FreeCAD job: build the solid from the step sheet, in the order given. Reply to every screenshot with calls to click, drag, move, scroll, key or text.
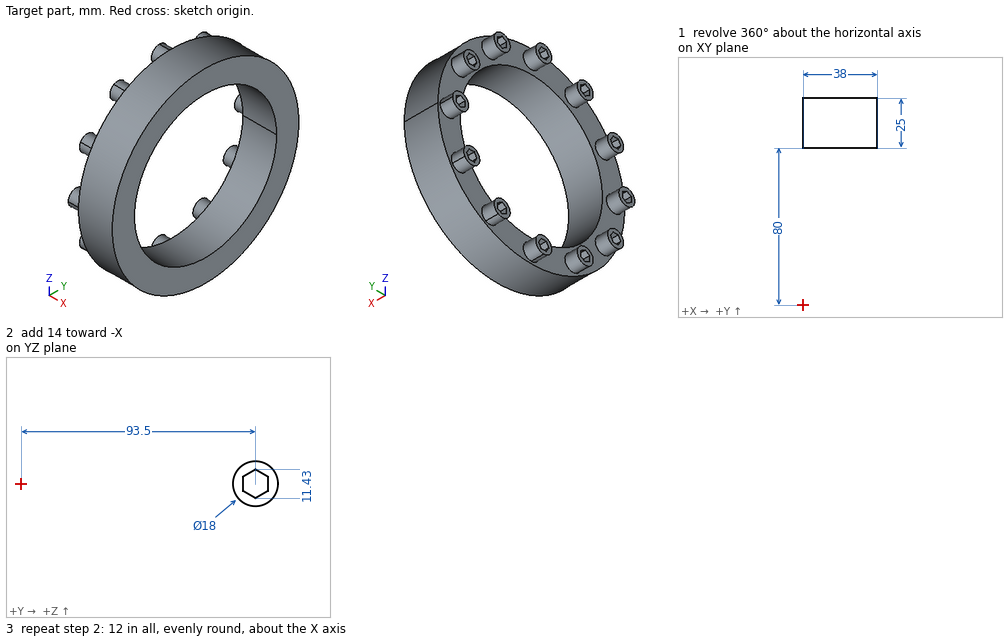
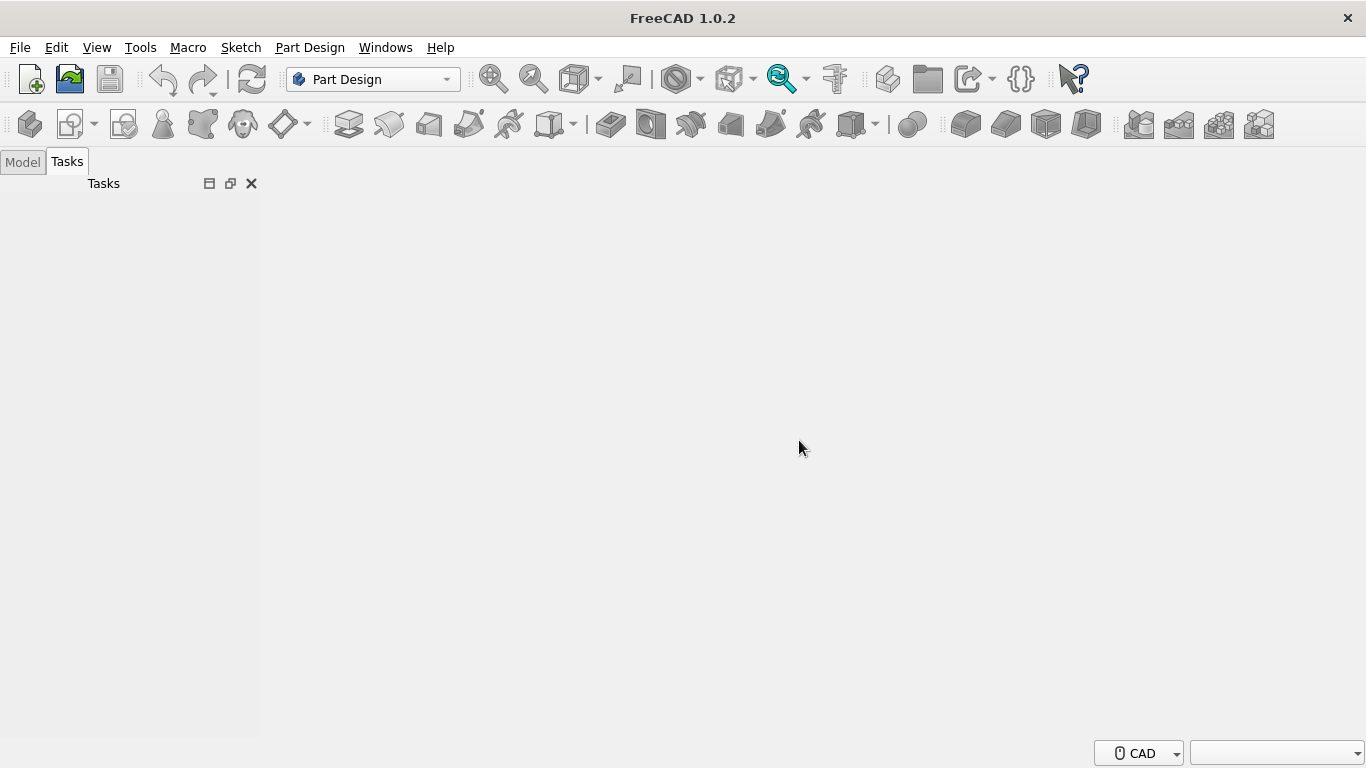
click(30, 80)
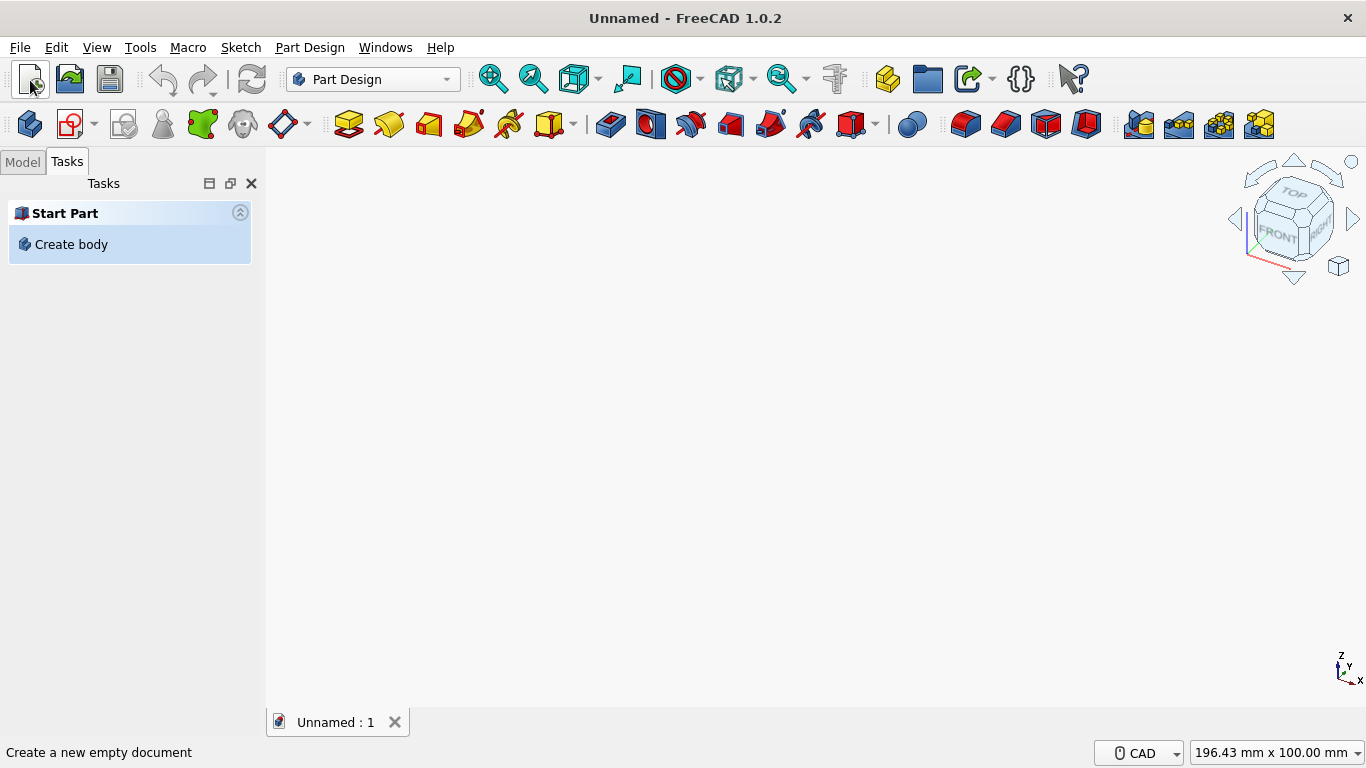
click(70, 124)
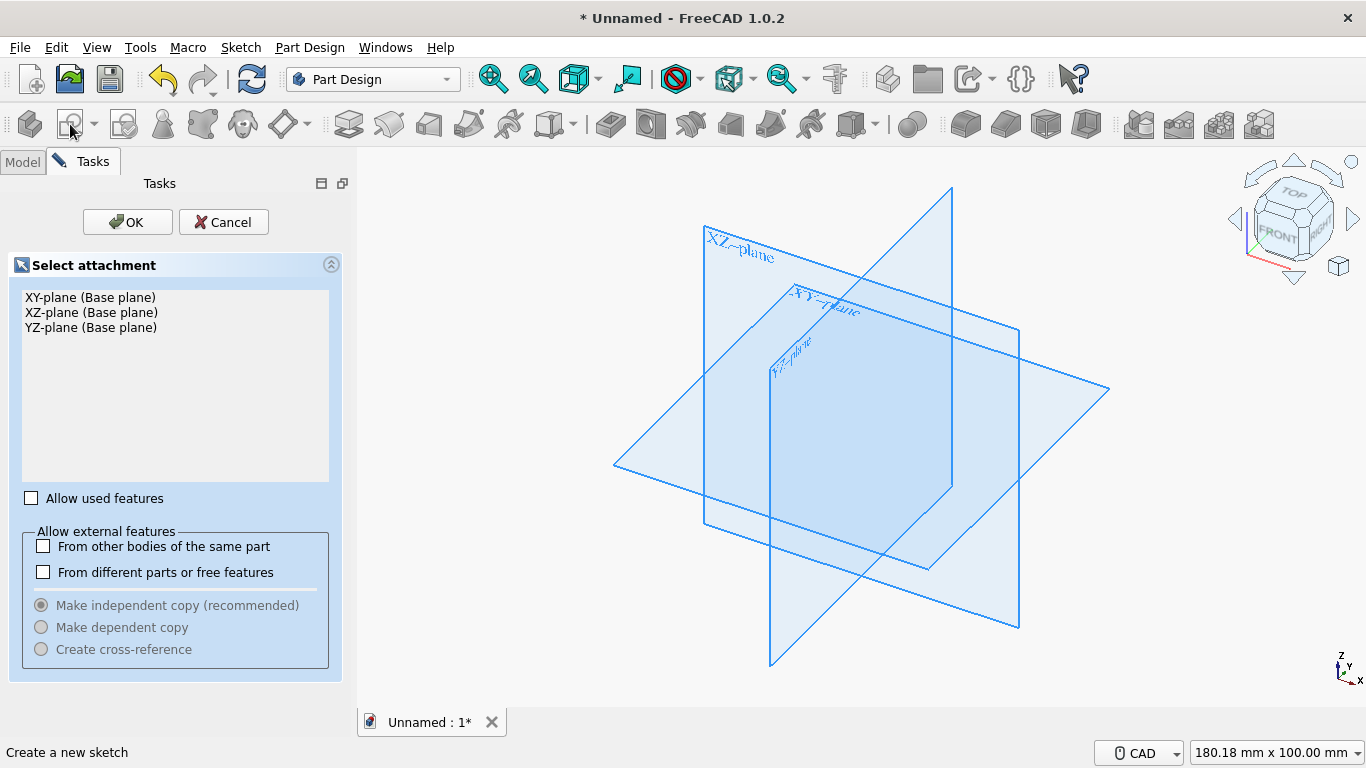
click(82, 298)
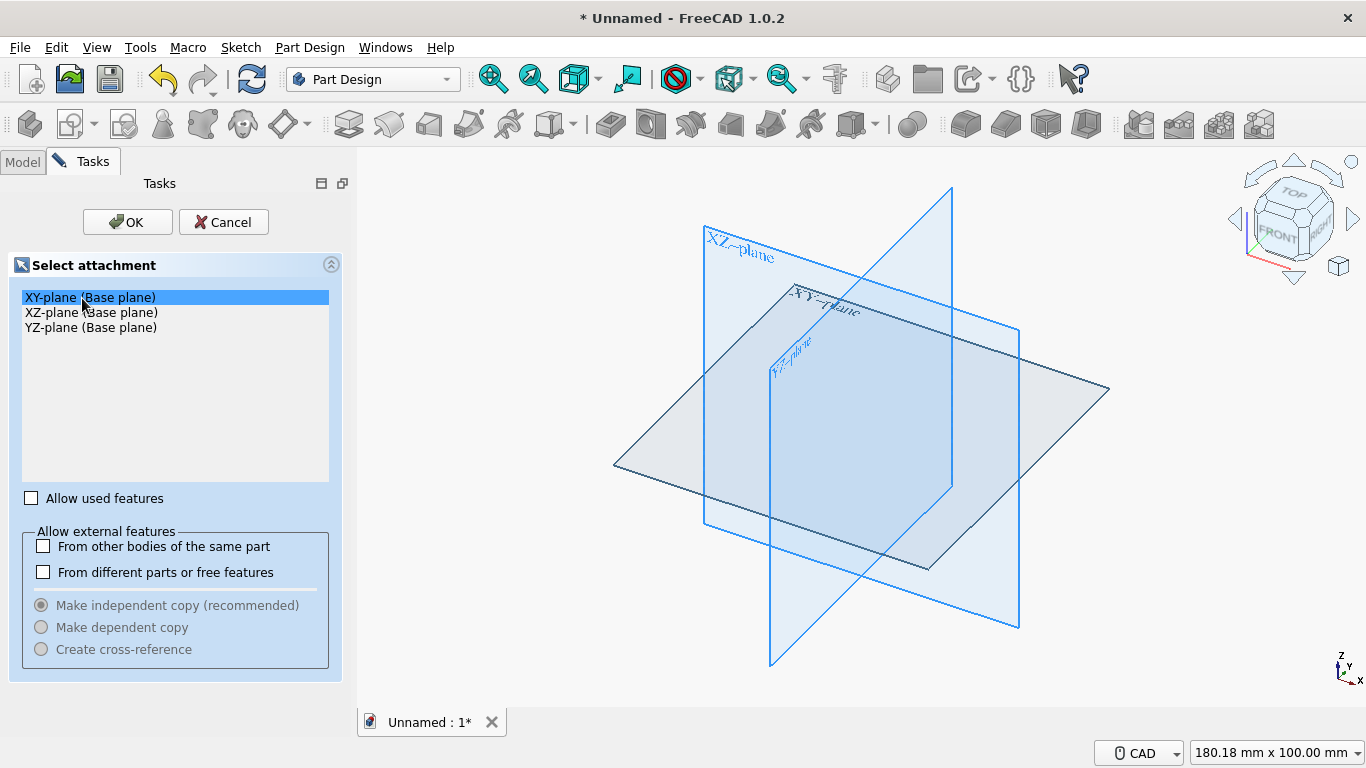
click(128, 222)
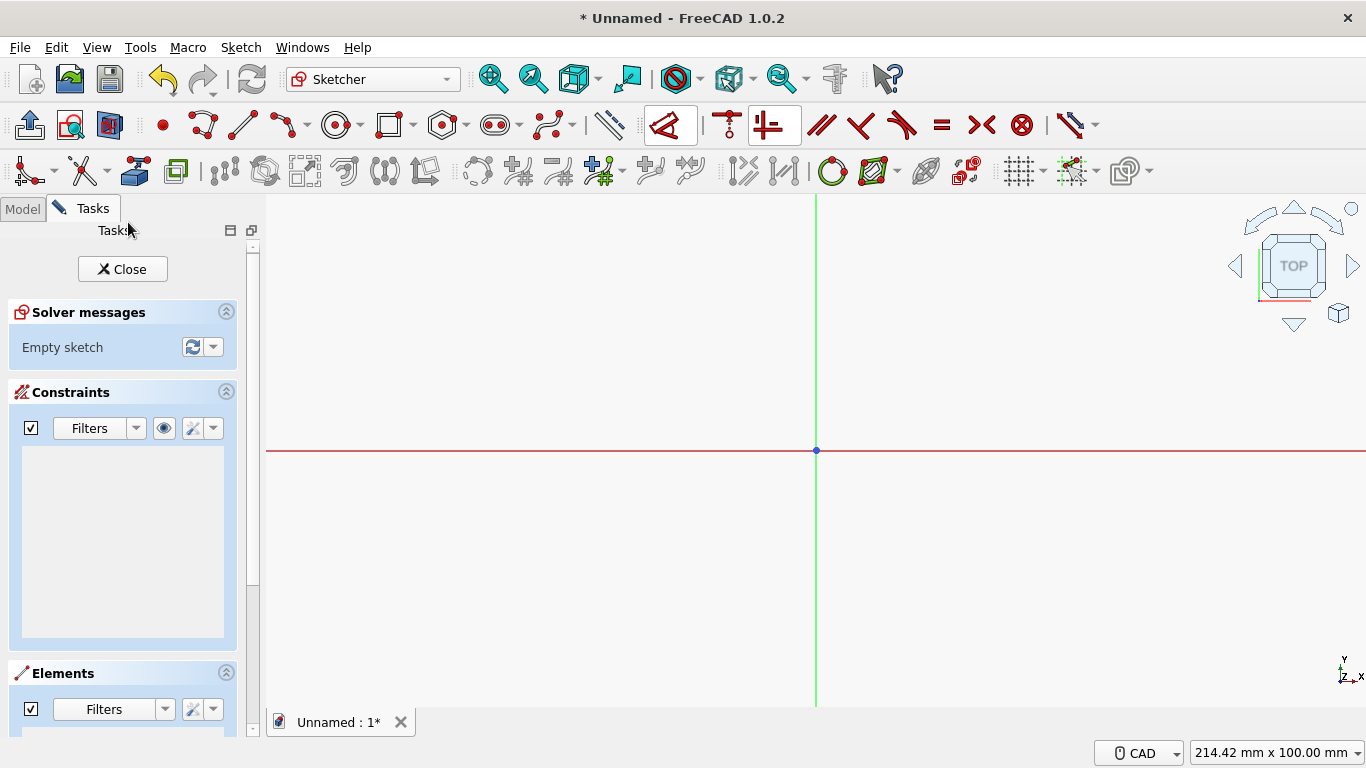
scroll(748, 450, down, 5)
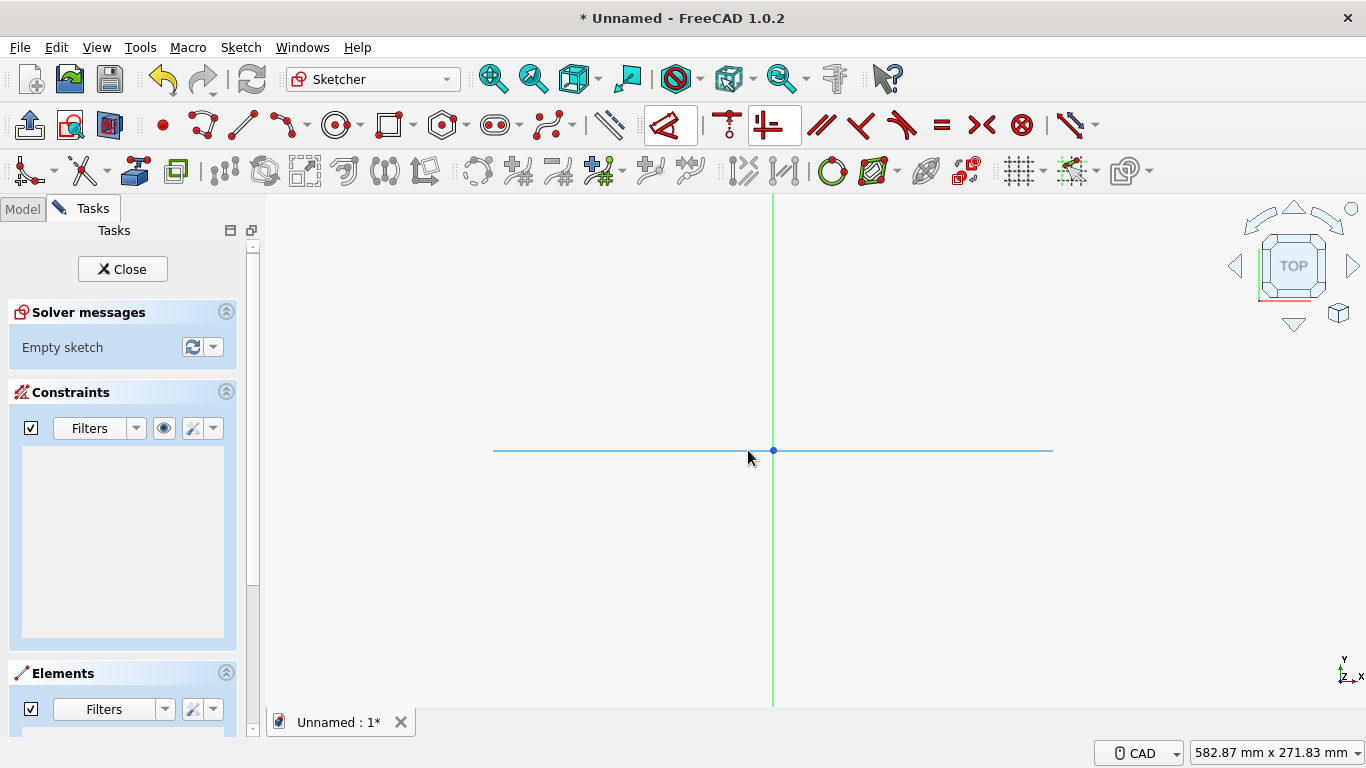
scroll(819, 249, up, 10)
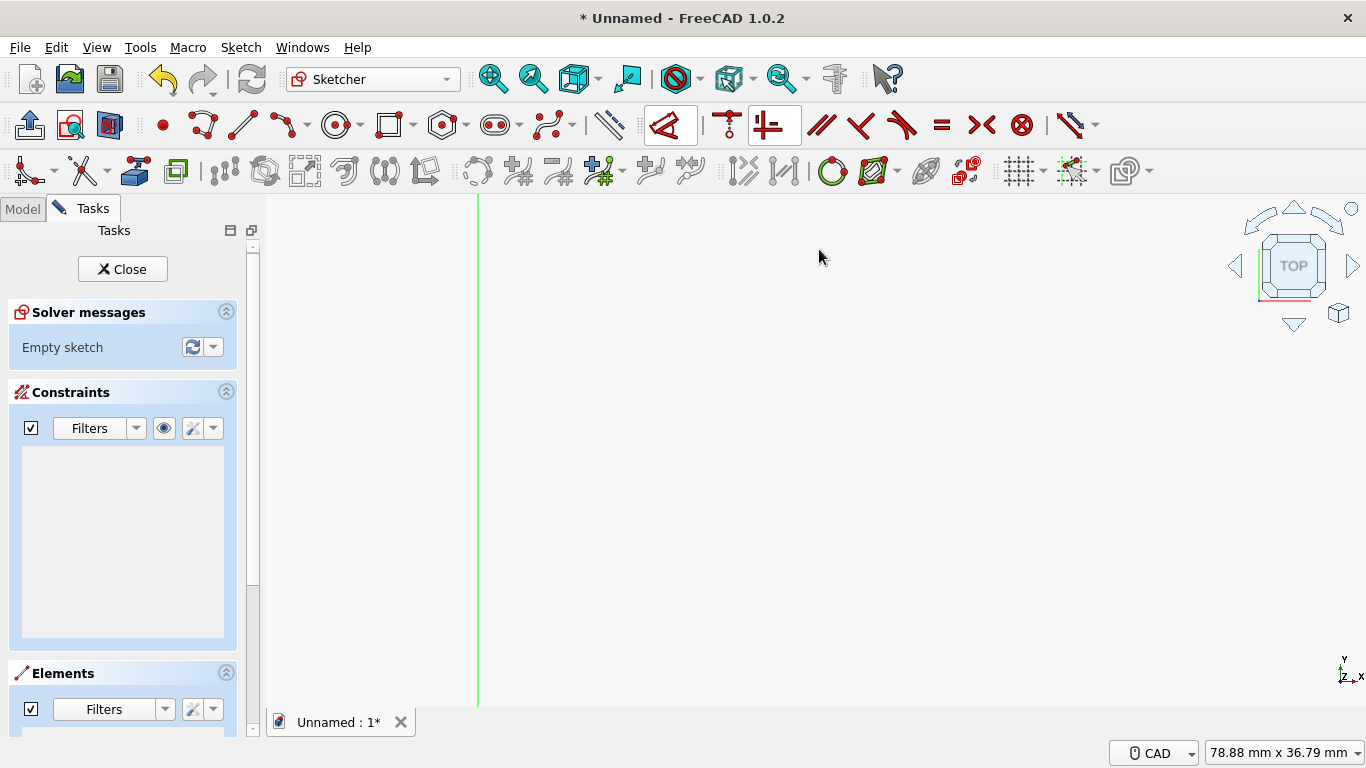
click(390, 126)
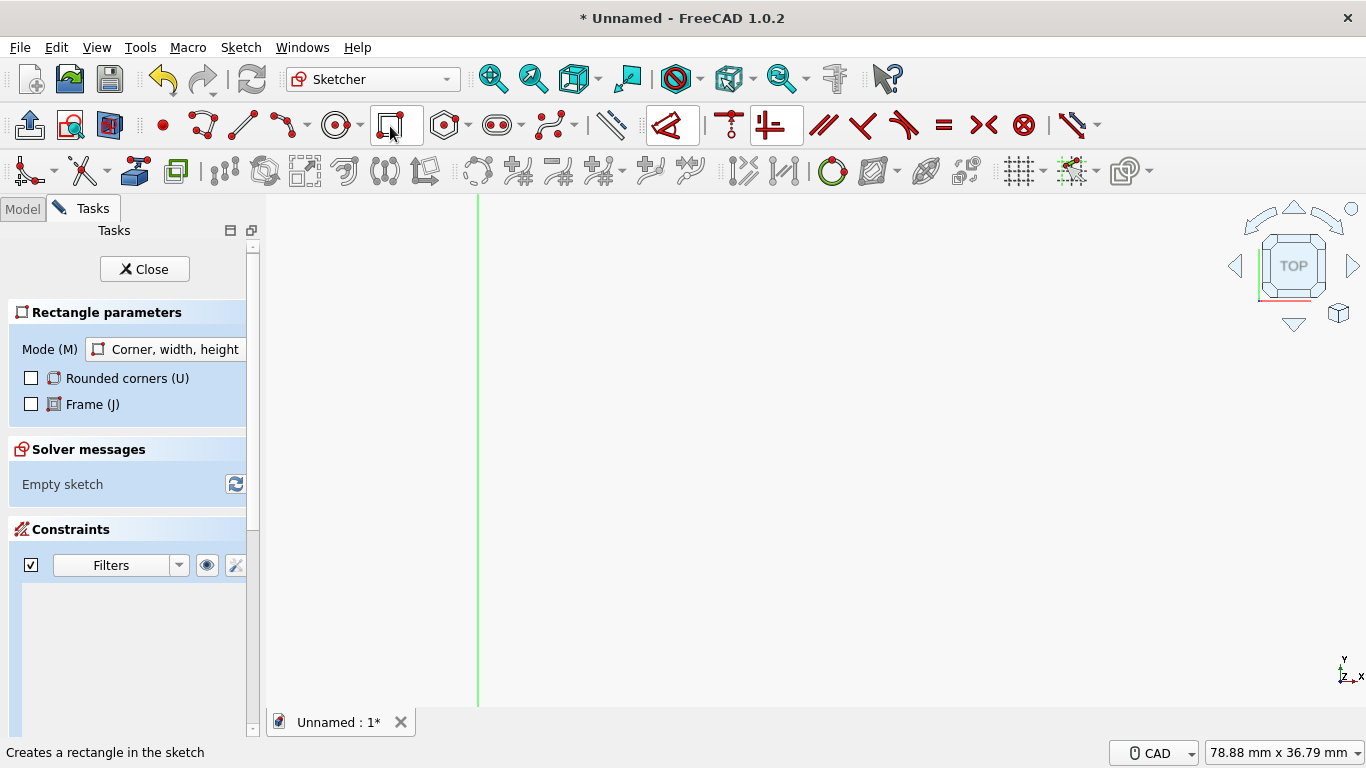
click(478, 273)
move(1008, 622)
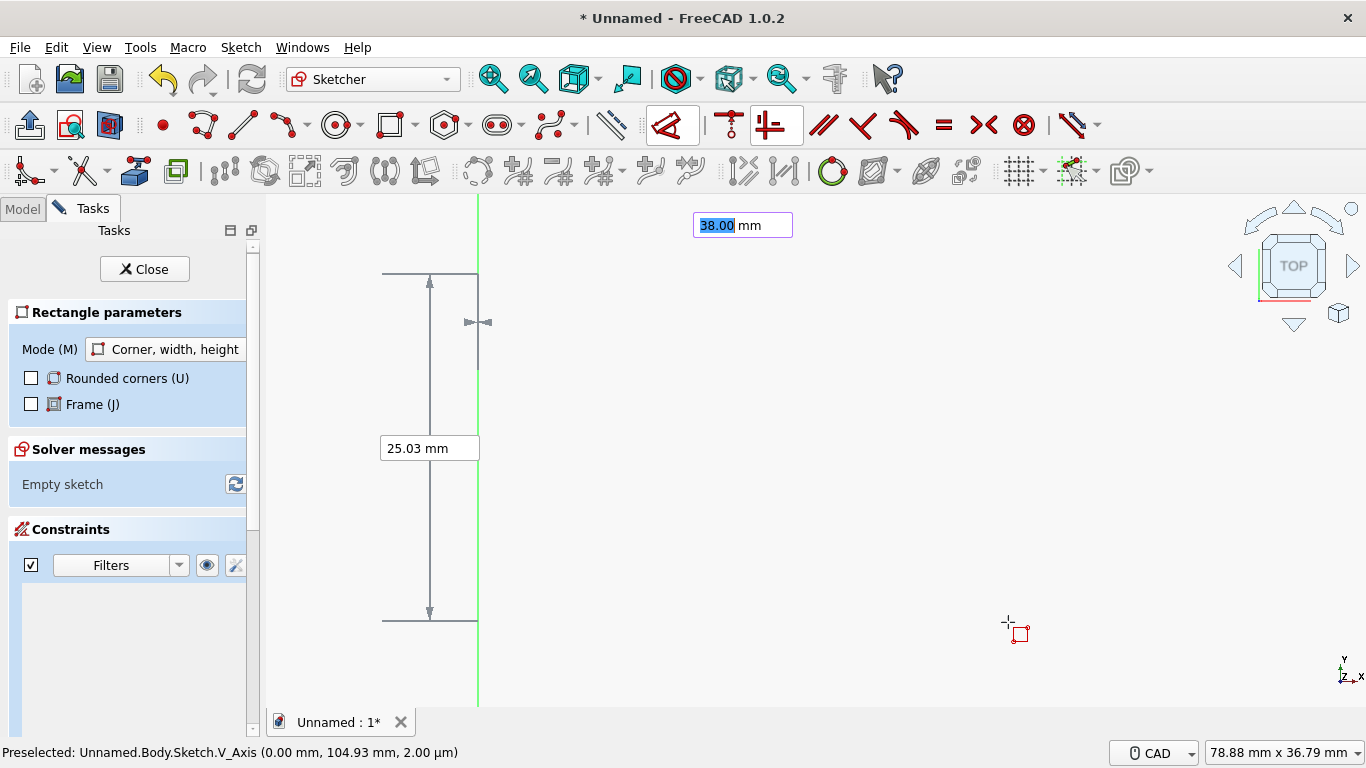
text(38)
key(Tab)
text(25)
key(Return)
key(Escape)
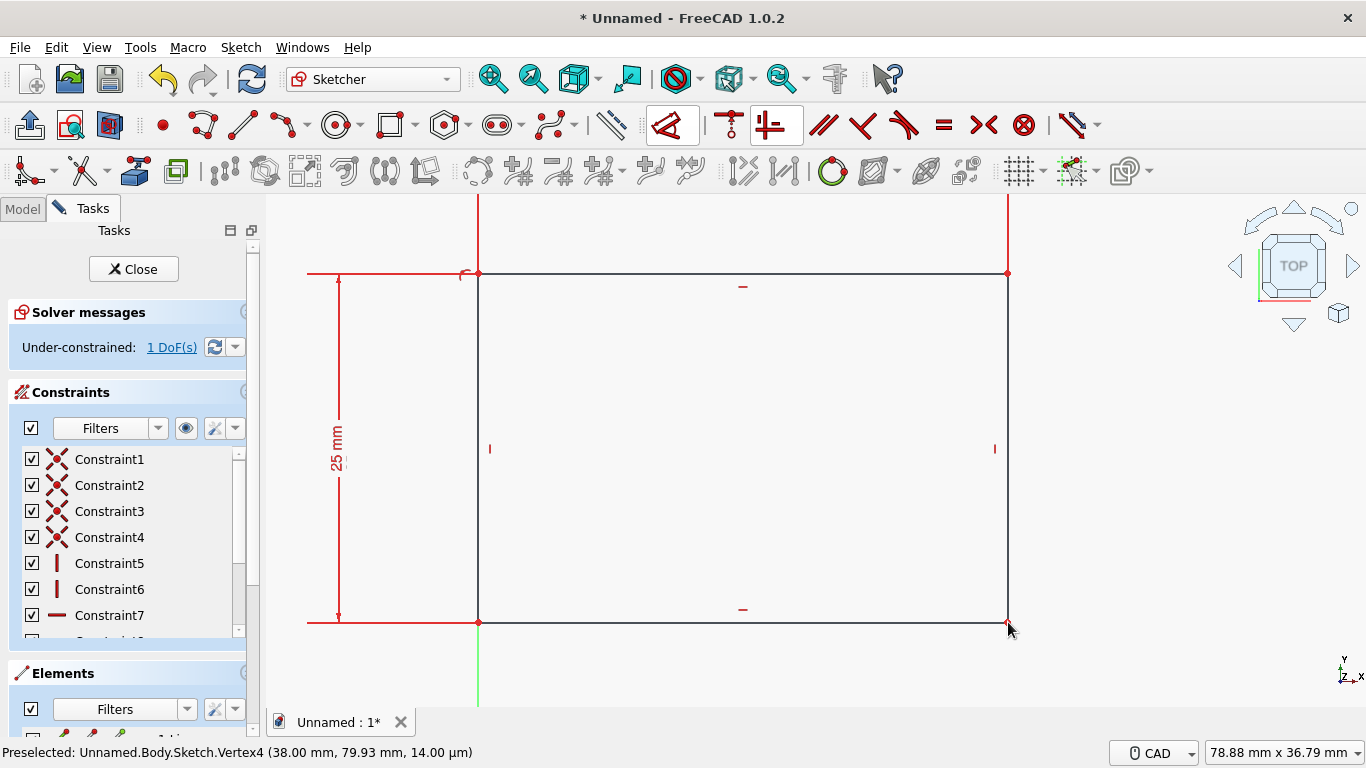
key(d)